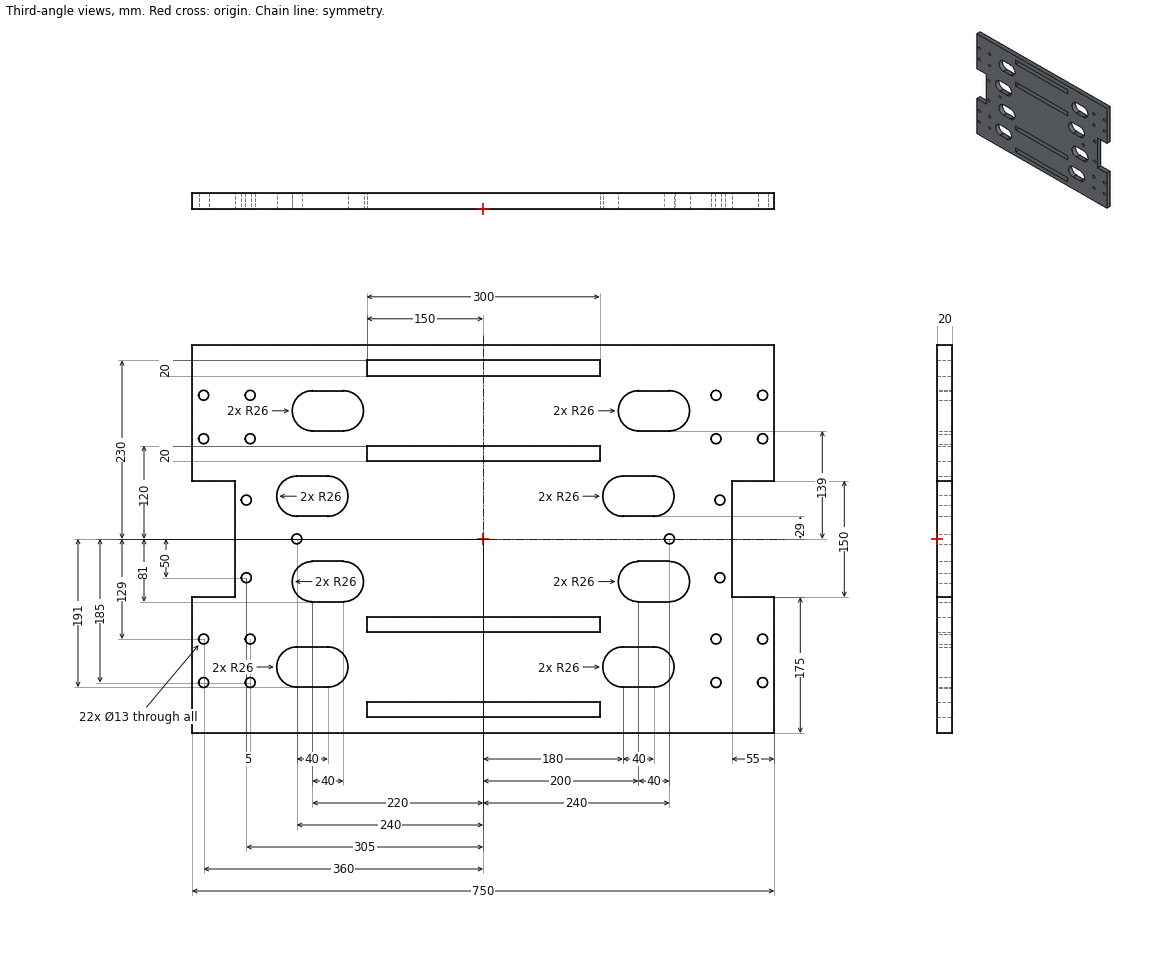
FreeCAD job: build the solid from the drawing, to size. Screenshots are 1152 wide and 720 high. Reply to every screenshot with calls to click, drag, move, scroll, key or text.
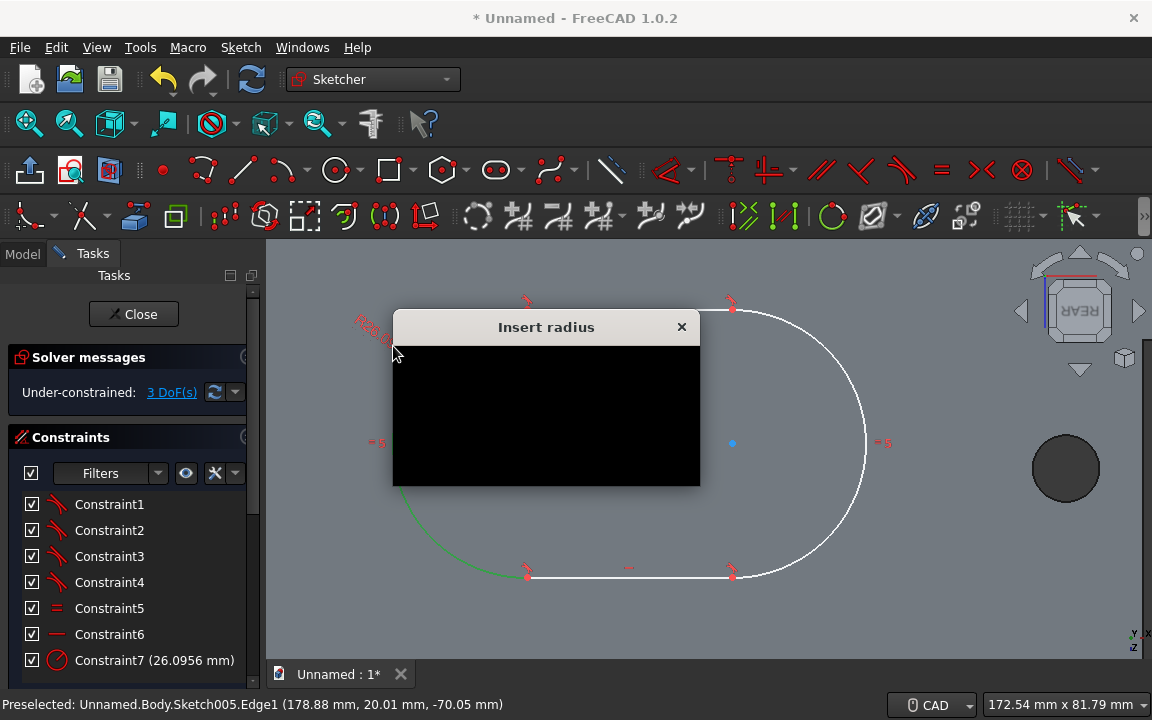
text(26)
key(Return)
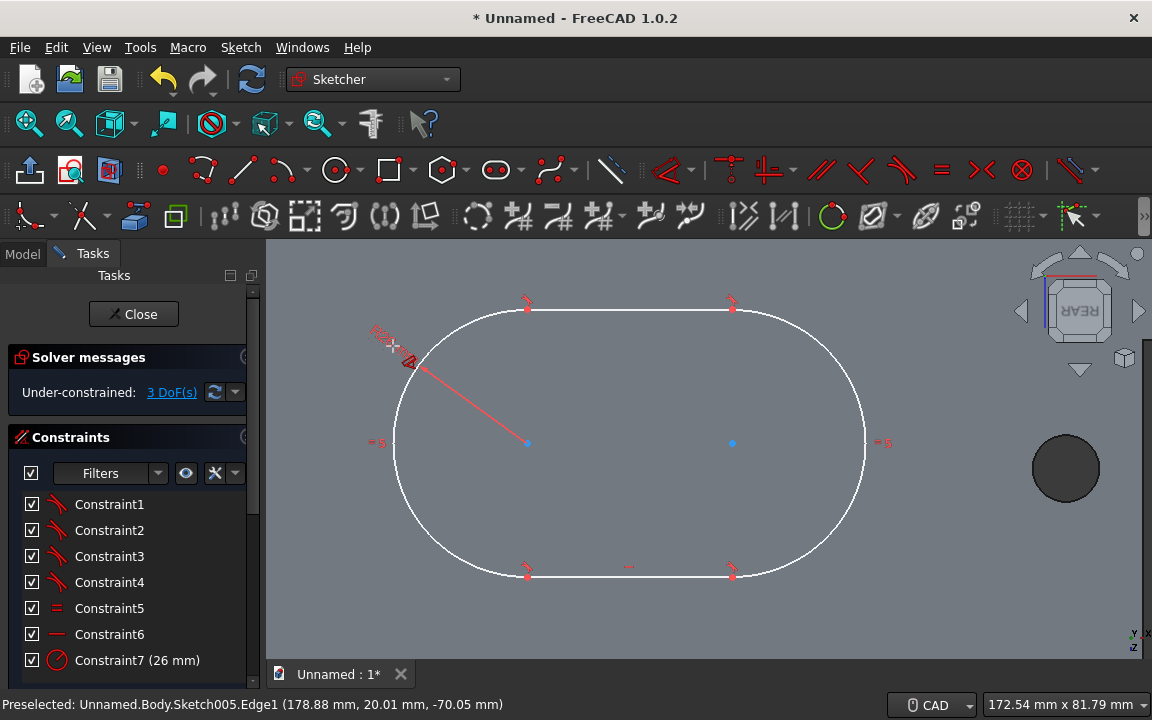
click(589, 310)
click(629, 276)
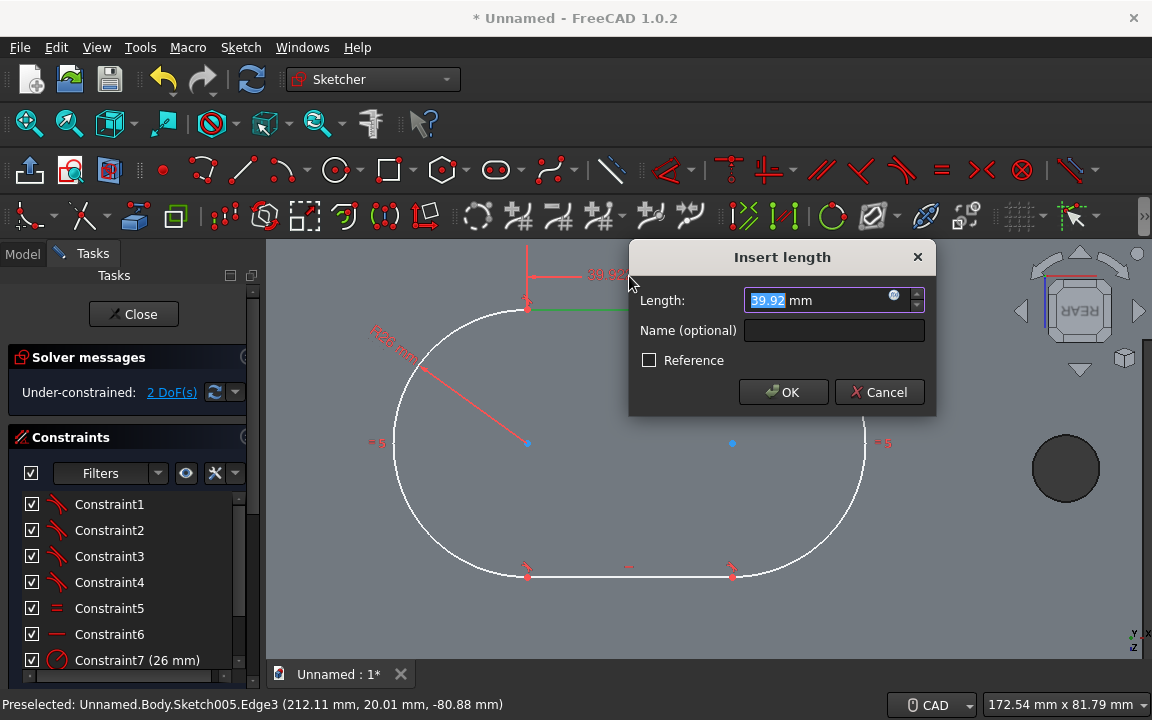
text(40)
key(Return)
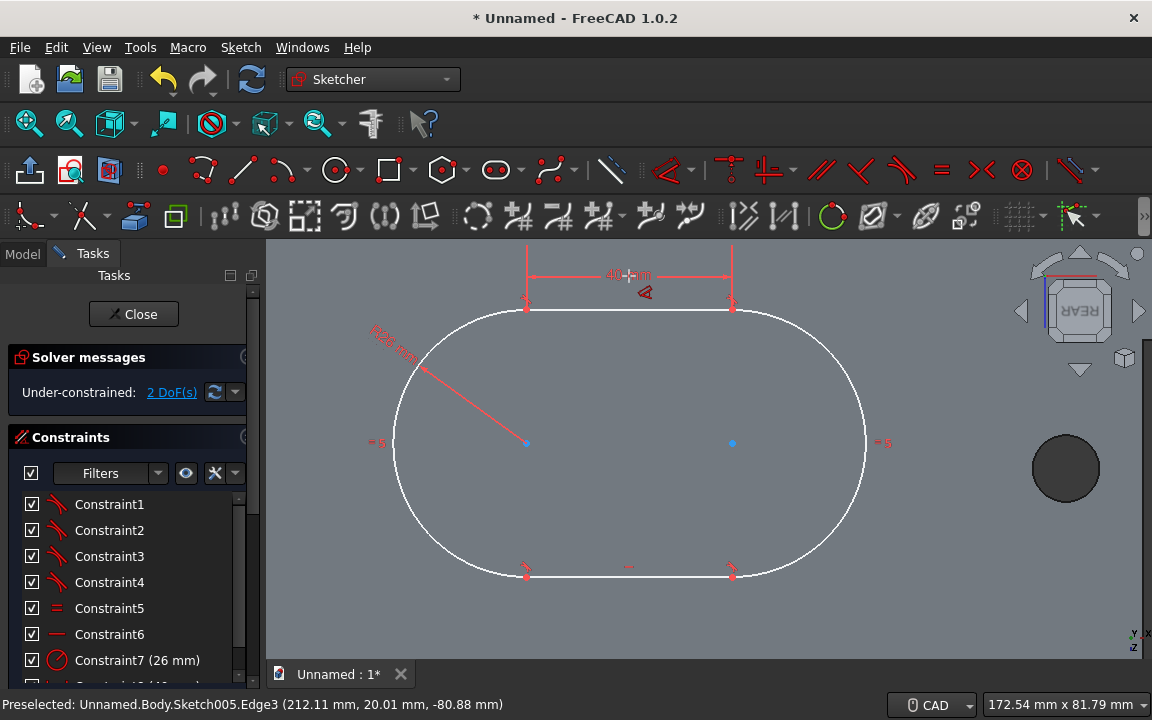
click(527, 310)
click(561, 470)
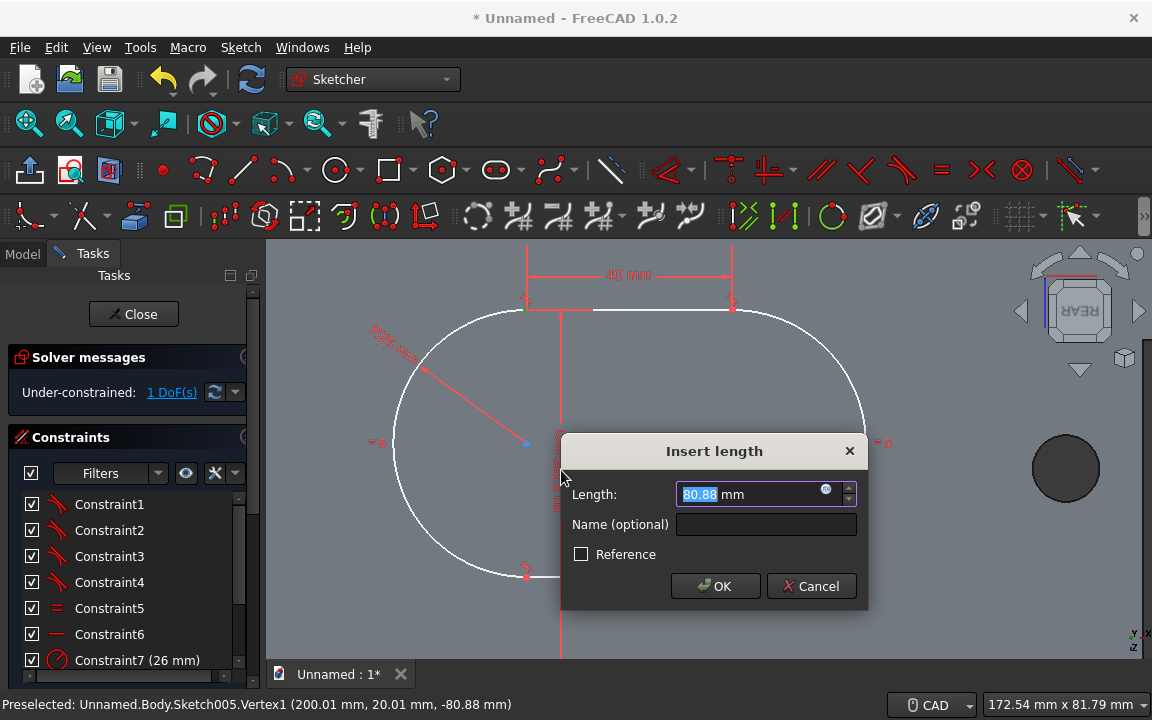
text(81)
key(Return)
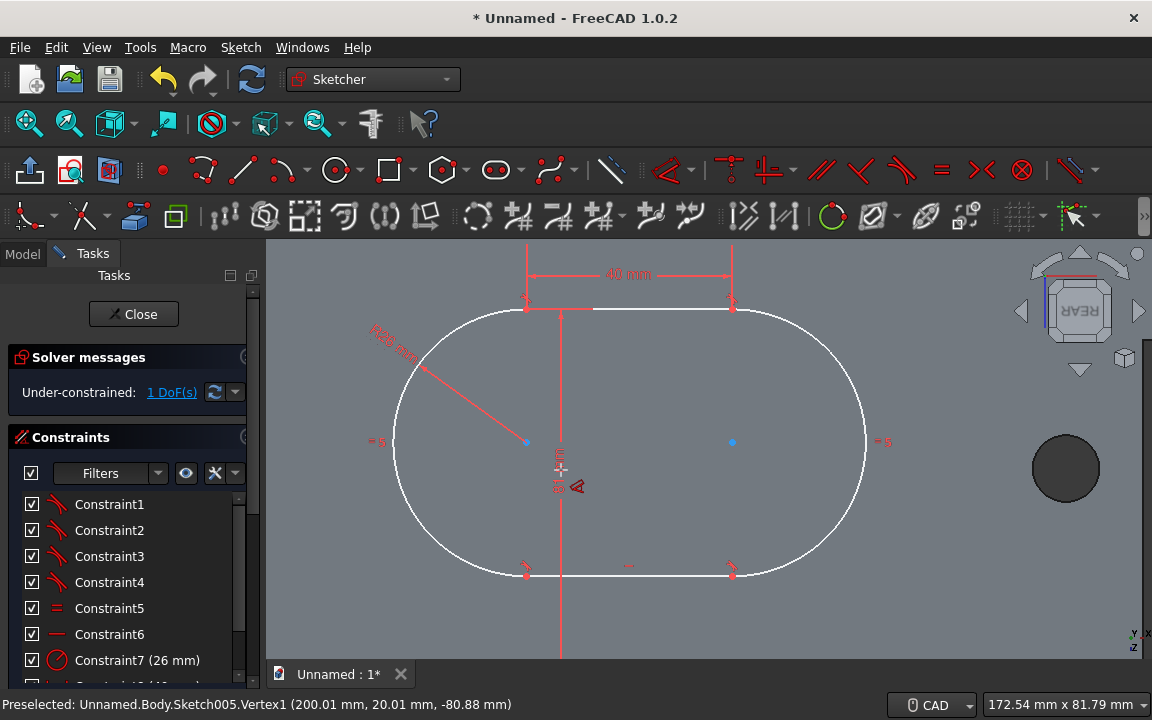
click(527, 309)
click(410, 275)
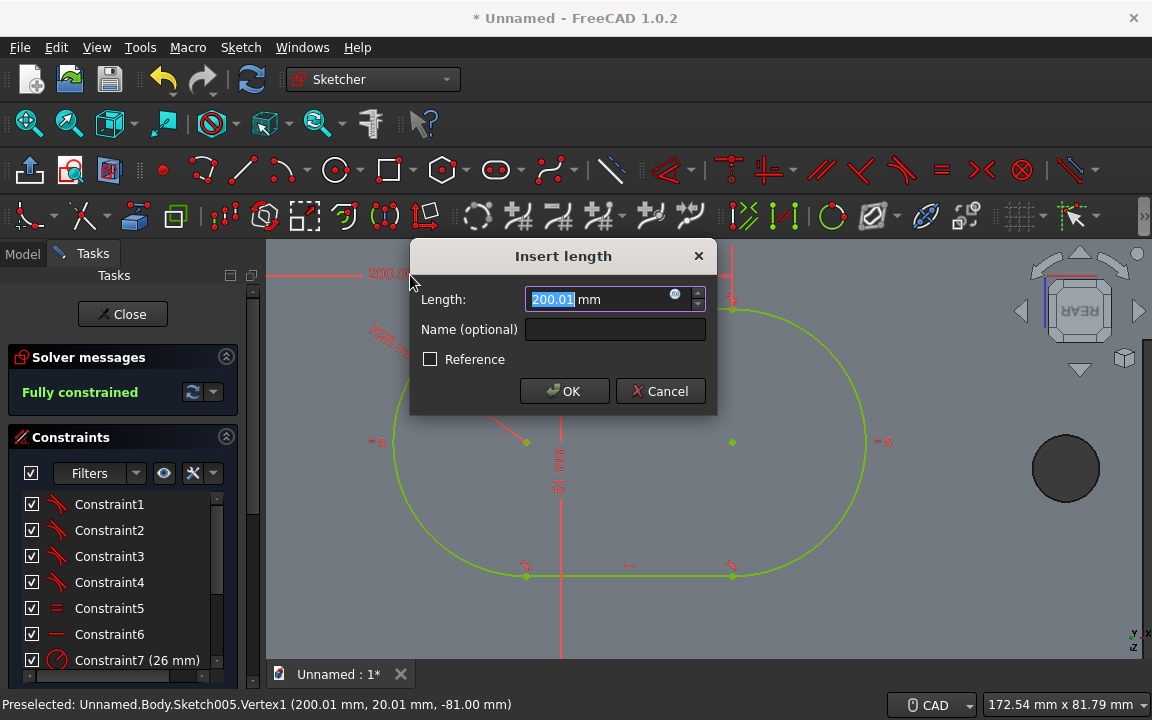
text(200)
key(Return)
key(Escape)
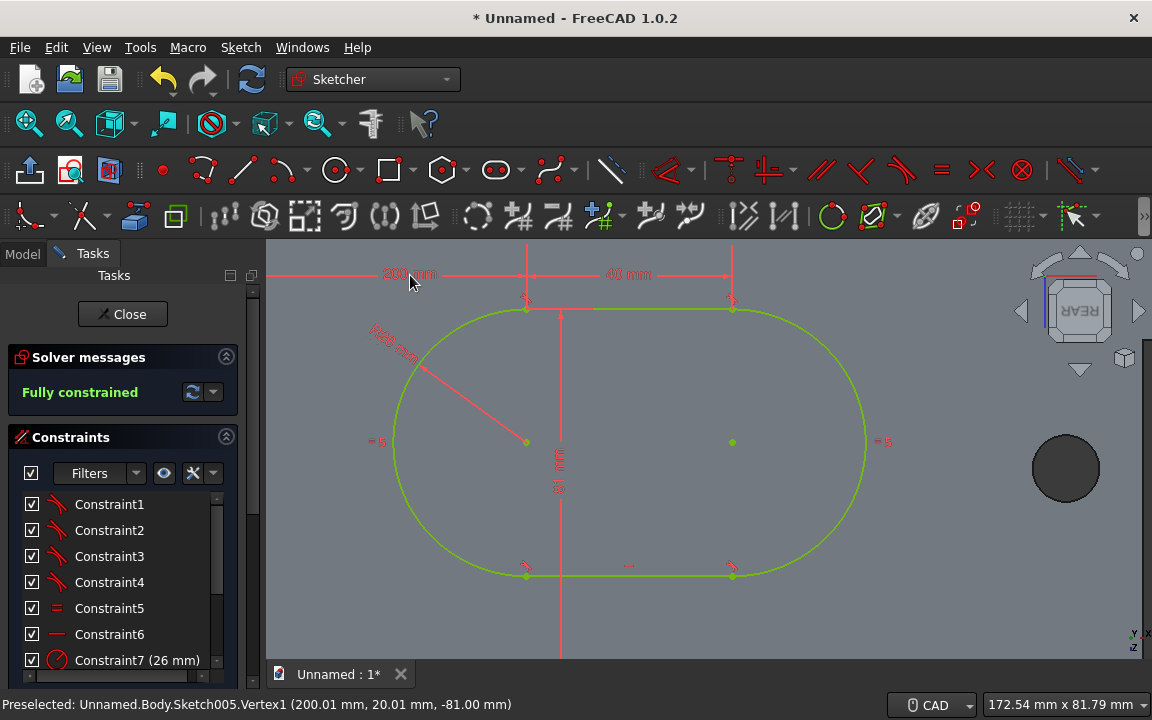
click(123, 314)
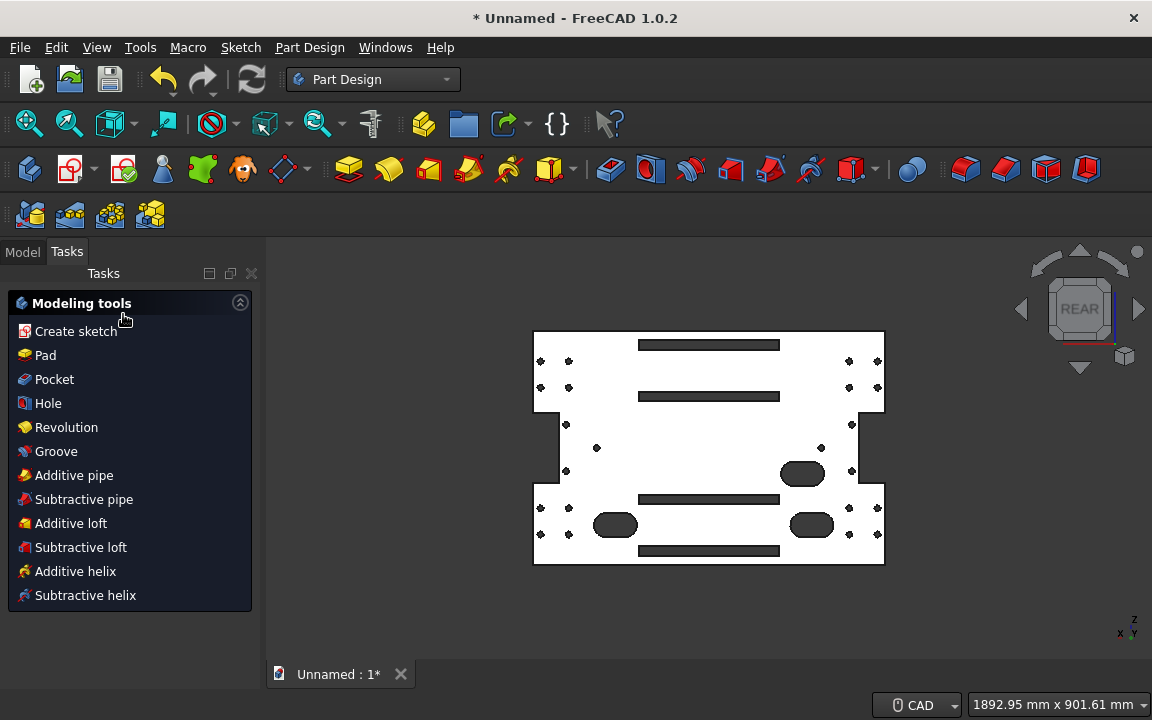
click(612, 170)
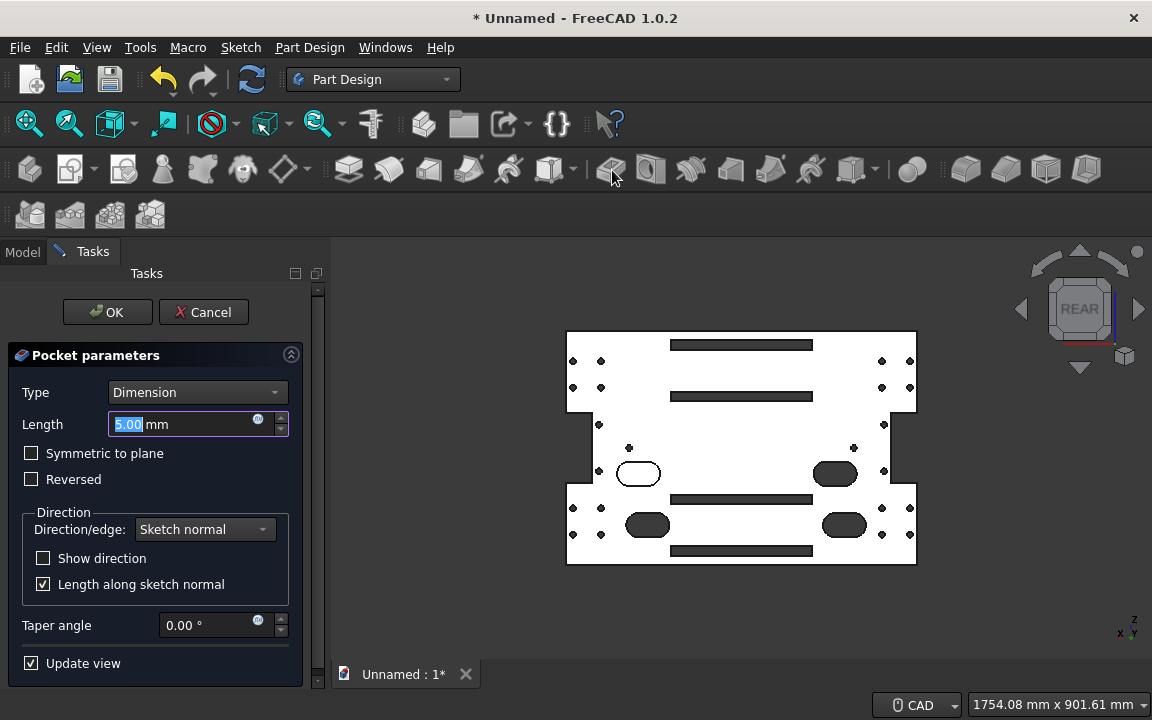
click(198, 392)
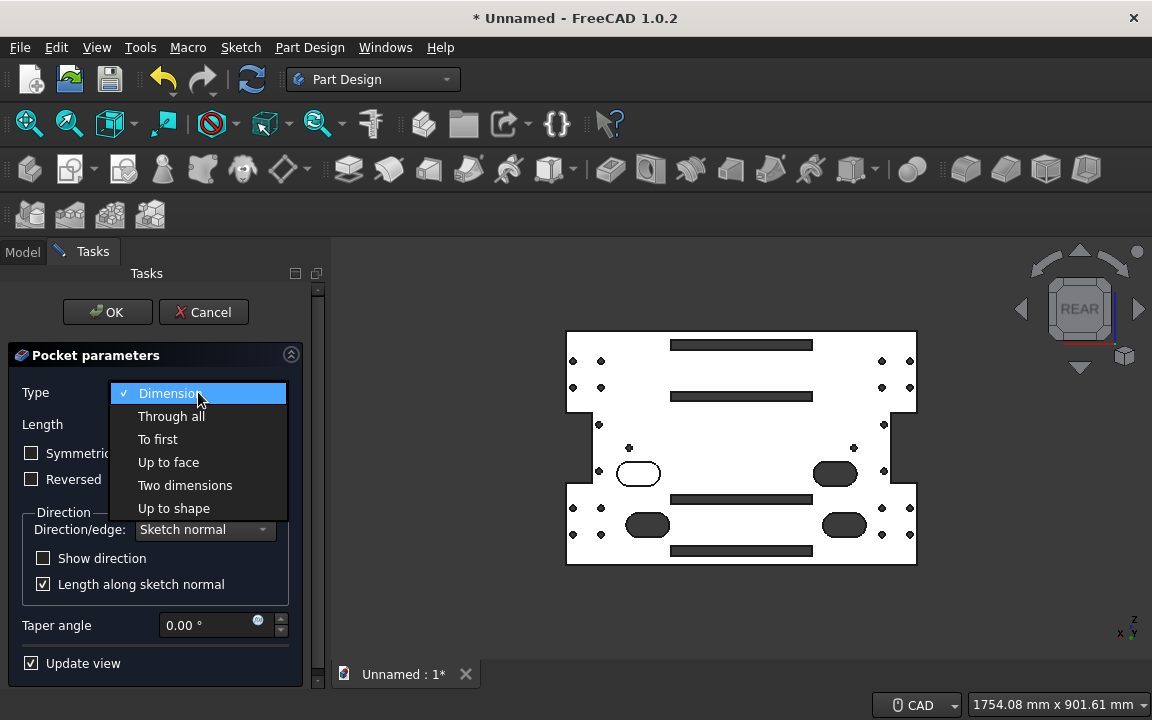
click(198, 440)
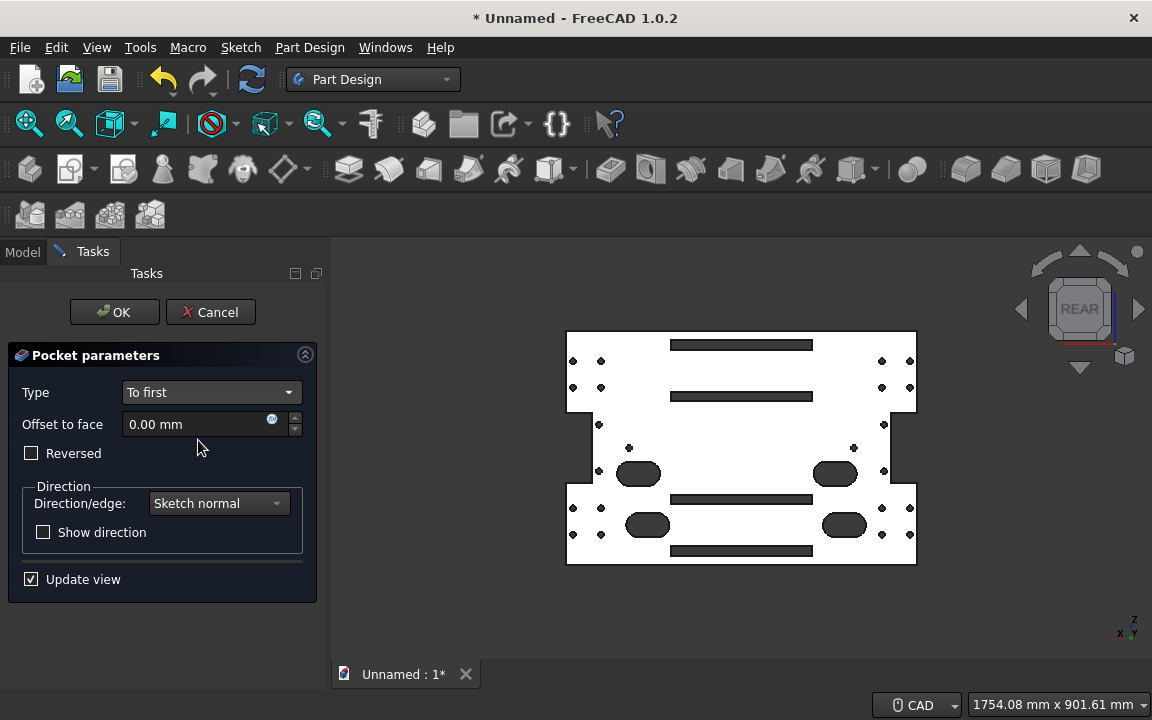
click(115, 312)